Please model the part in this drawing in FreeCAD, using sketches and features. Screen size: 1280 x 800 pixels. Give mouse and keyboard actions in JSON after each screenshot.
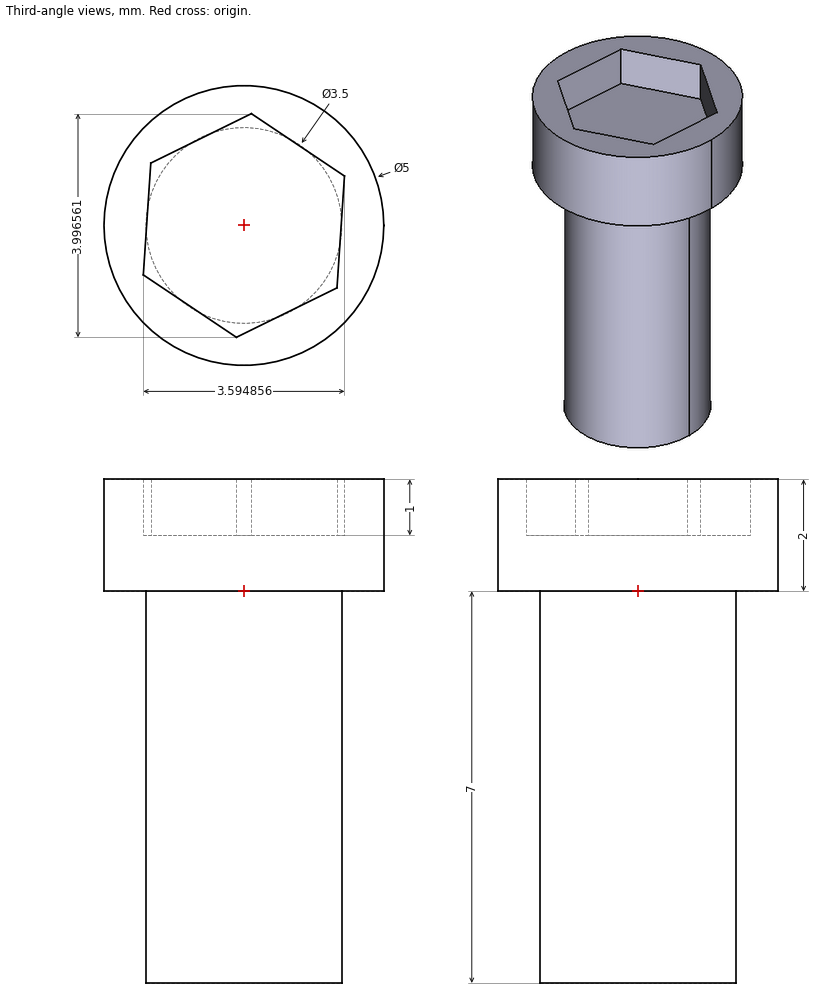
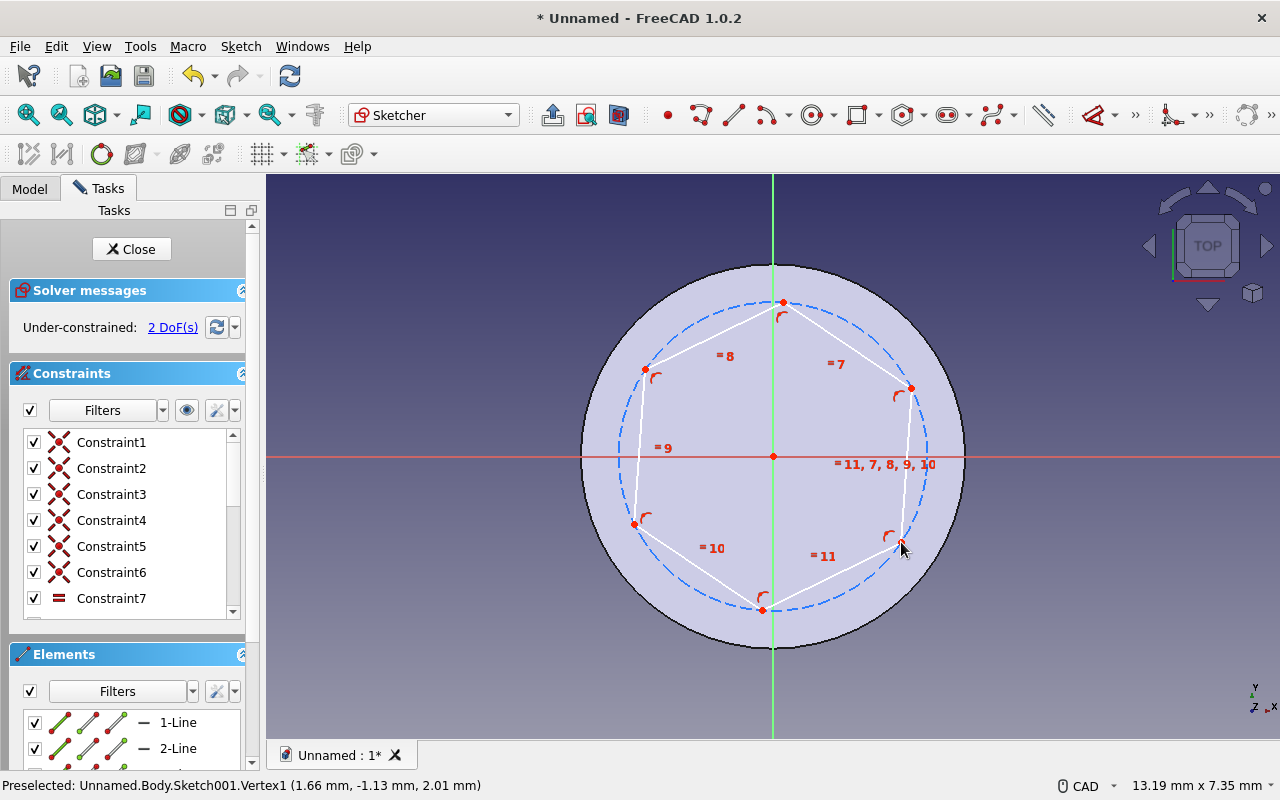
{"action": "left_click", "coordinate": [1092, 116]}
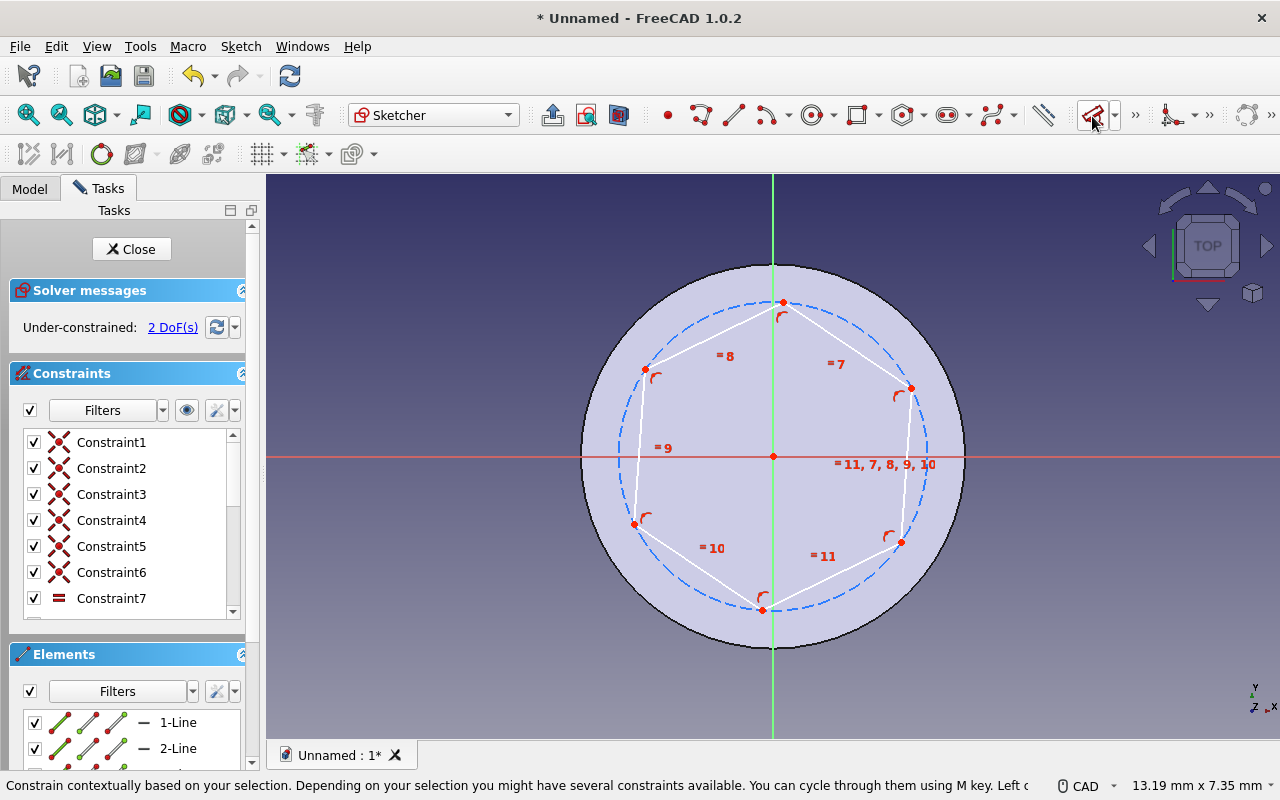
{"action": "left_click", "coordinate": [634, 524]}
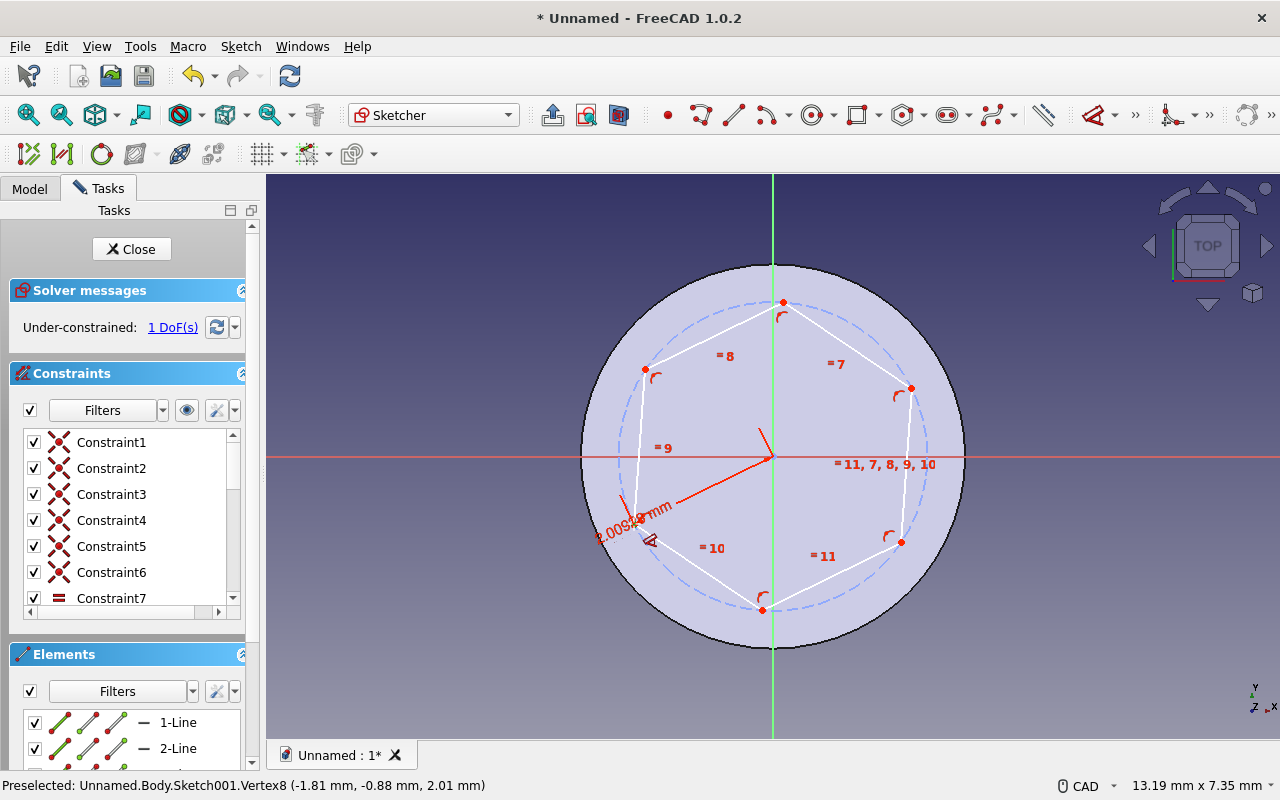
{"action": "left_click", "coordinate": [912, 389]}
{"action": "left_click", "coordinate": [709, 558]}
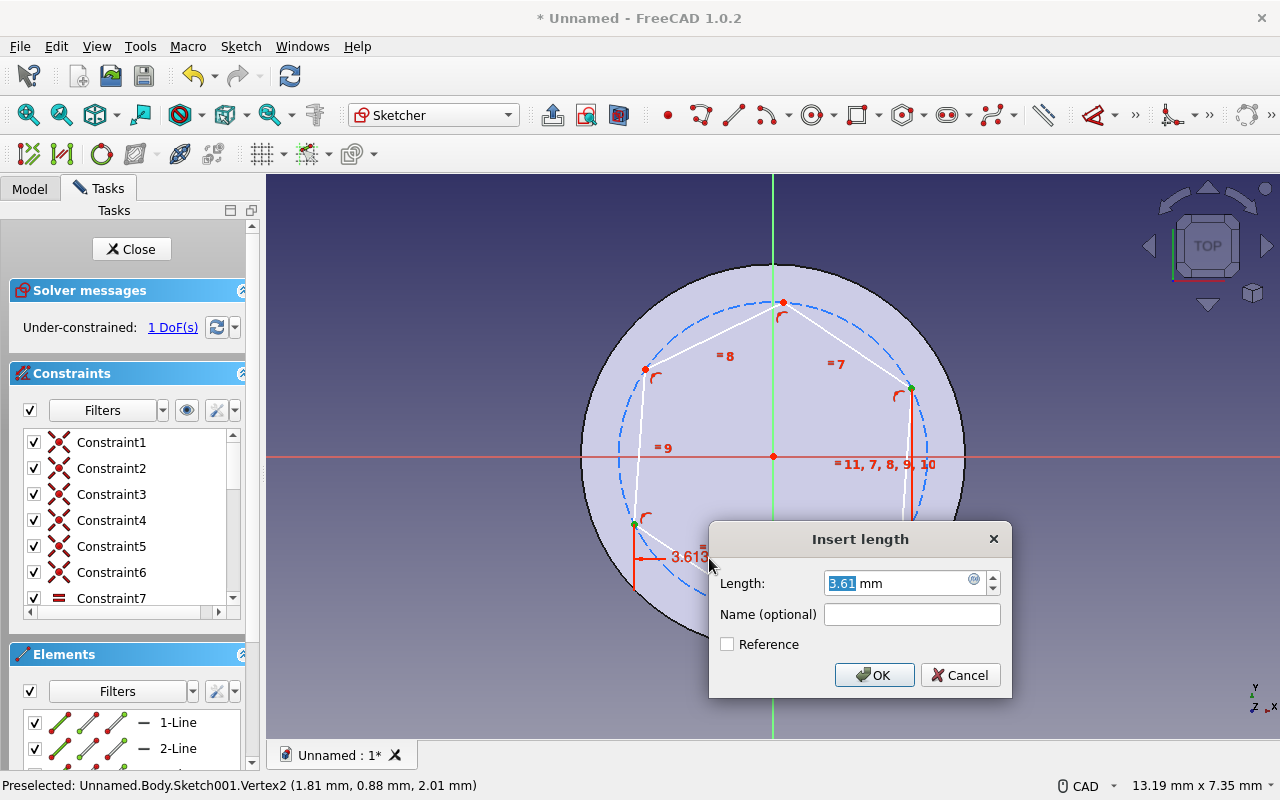
{"action": "type", "text": "3.594856"}
{"action": "key", "text": "Return"}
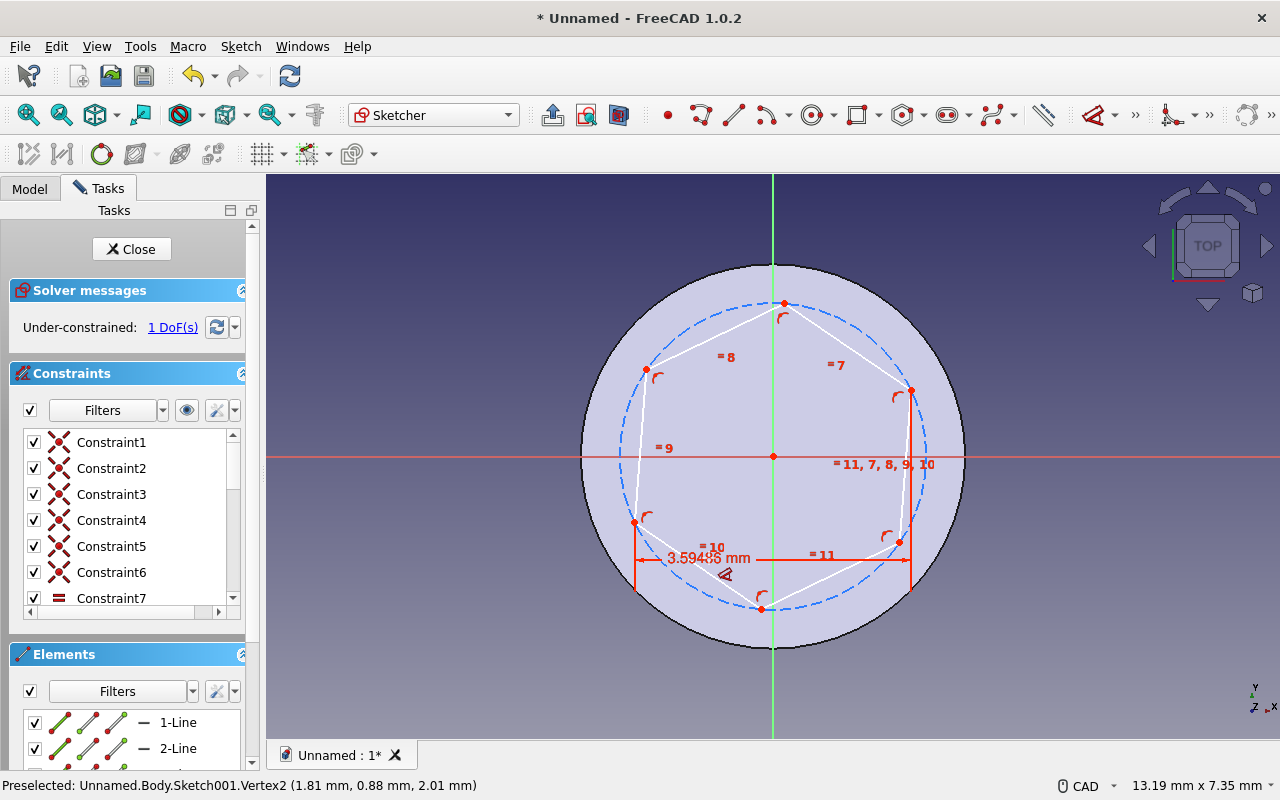
{"action": "left_click", "coordinate": [761, 609]}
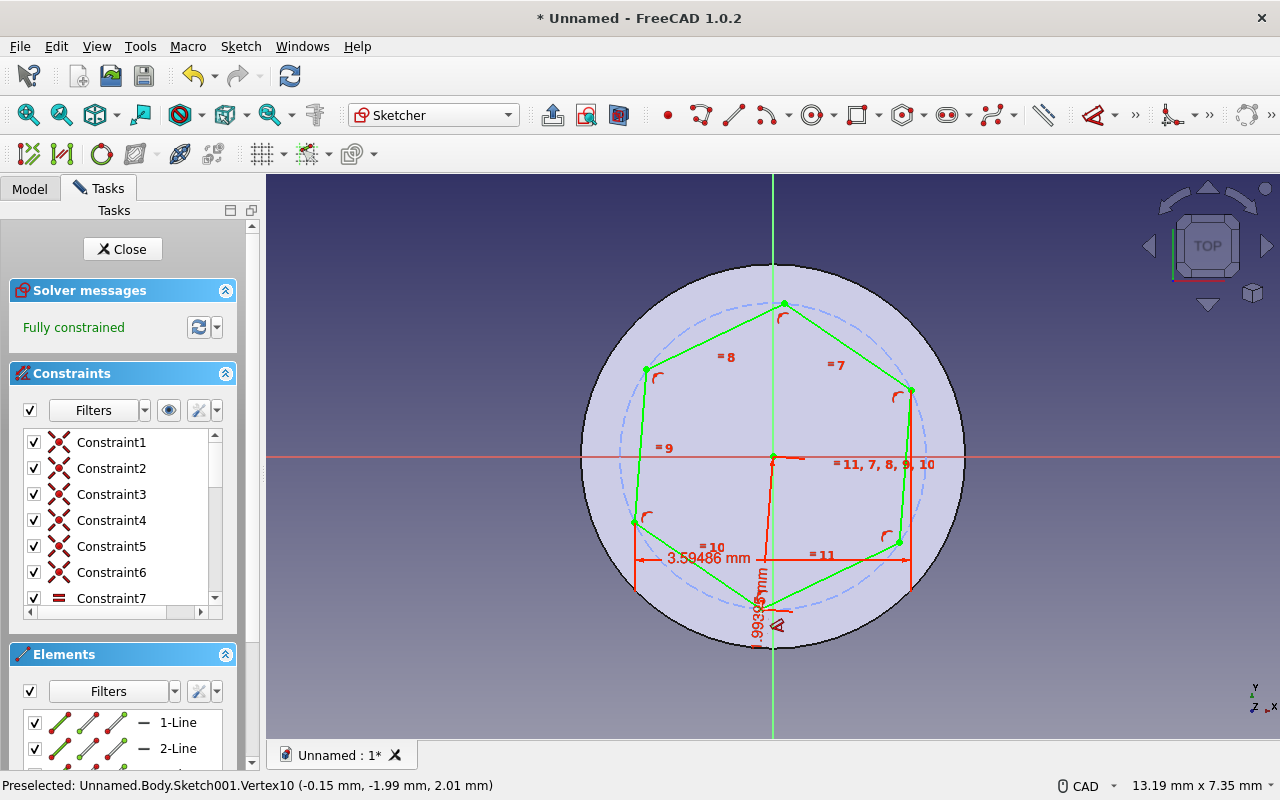
{"action": "left_click", "coordinate": [785, 304]}
{"action": "left_click", "coordinate": [819, 386]}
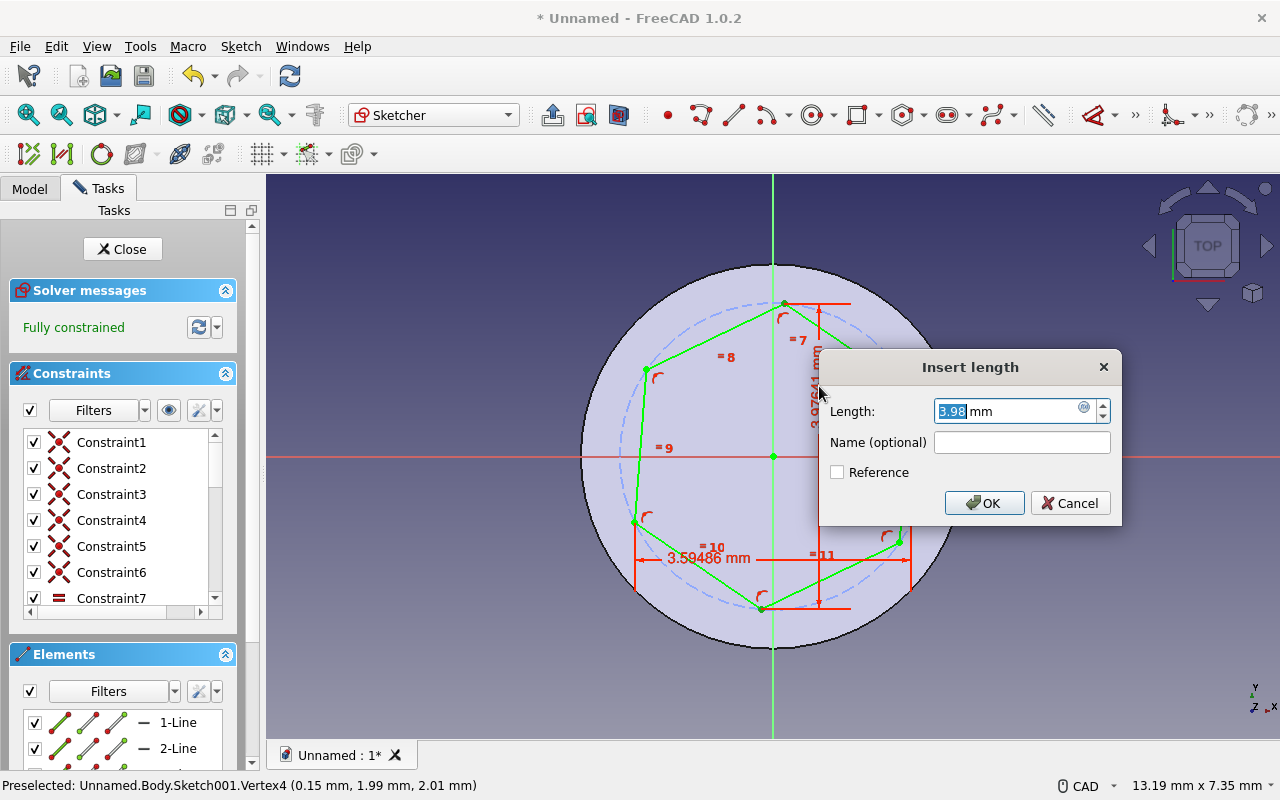
{"action": "type", "text": "3.996561"}
{"action": "key", "text": "Return"}
{"action": "key", "text": "Escape"}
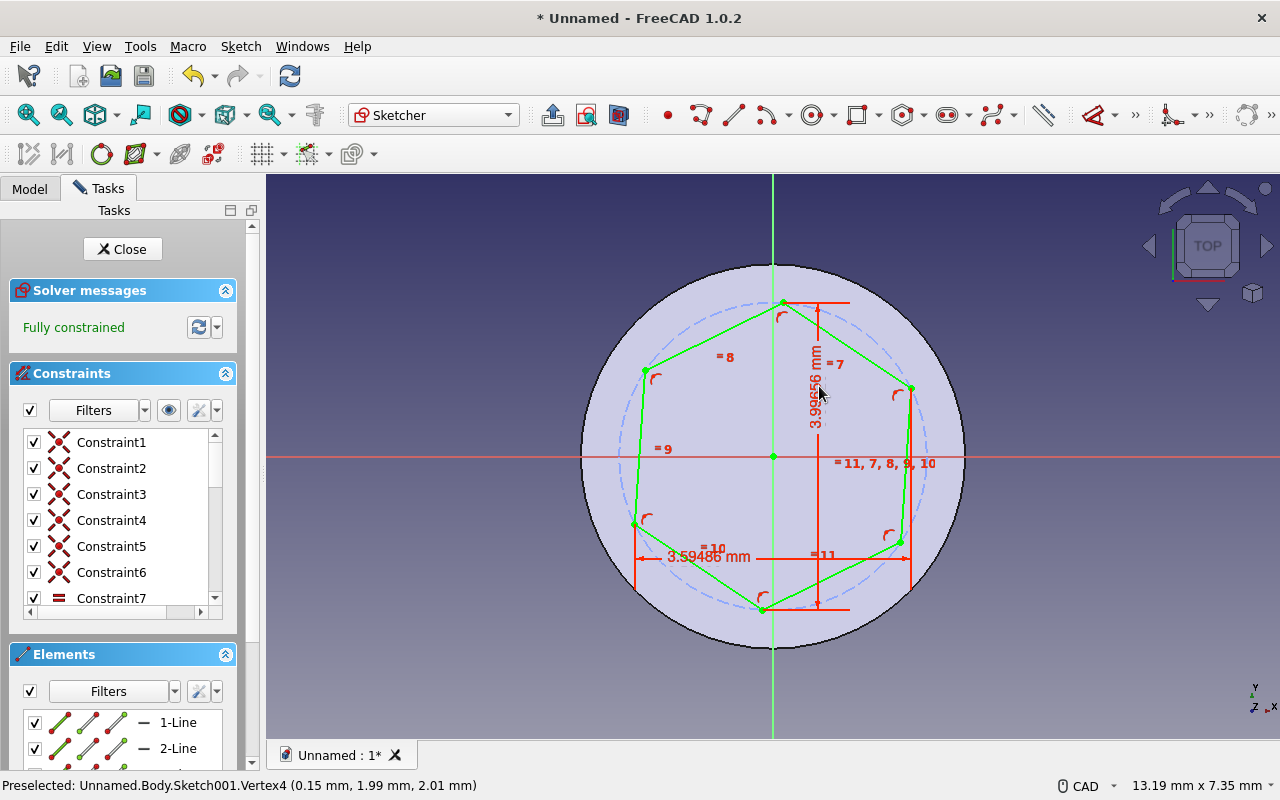
{"action": "left_click", "coordinate": [123, 249]}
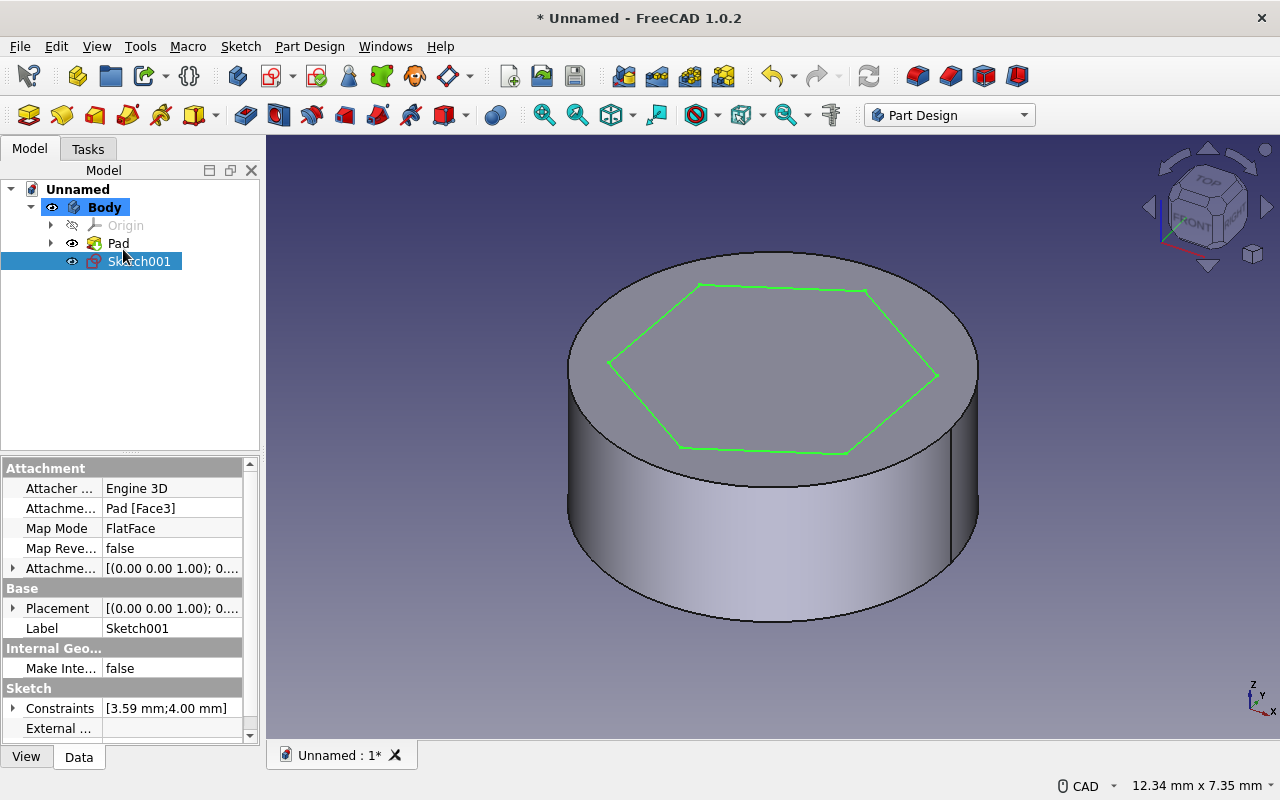
{"action": "left_click", "coordinate": [246, 116]}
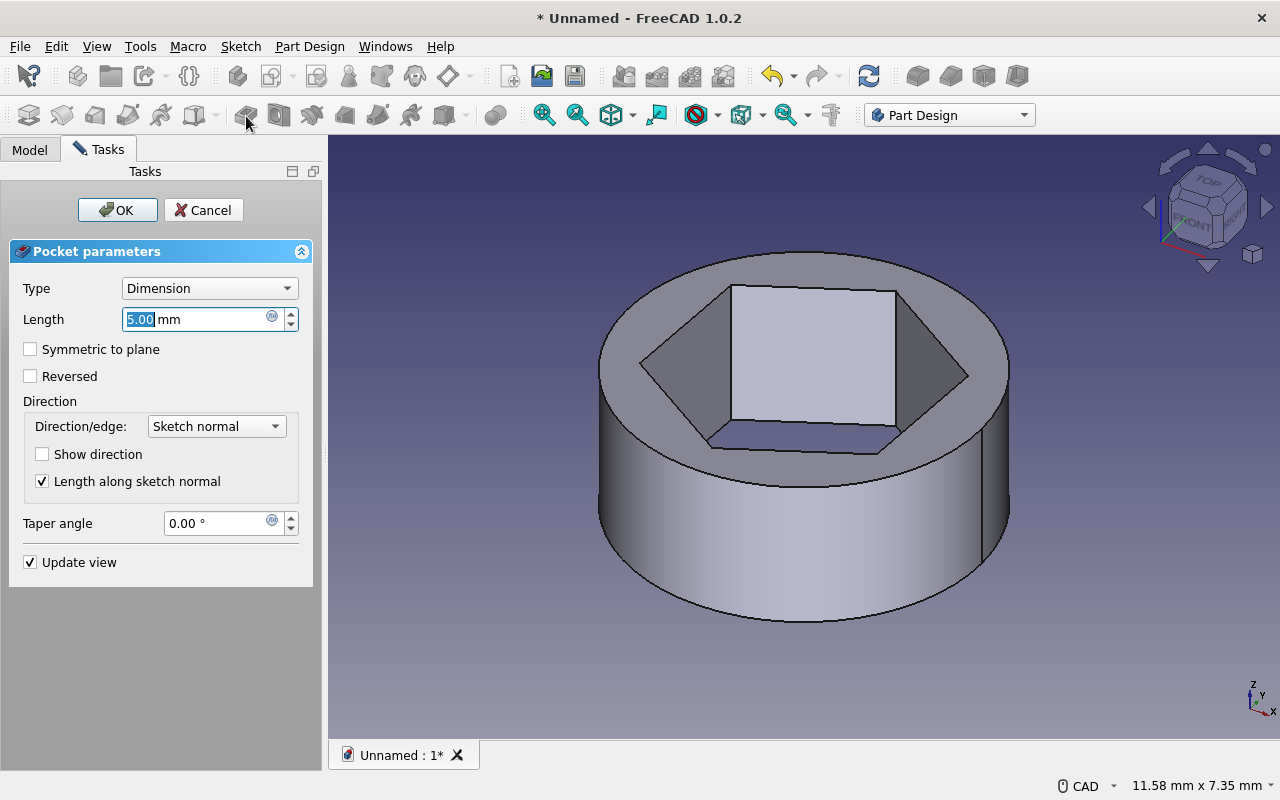
{"action": "type", "text": "1"}
{"action": "key", "text": "Tab"}